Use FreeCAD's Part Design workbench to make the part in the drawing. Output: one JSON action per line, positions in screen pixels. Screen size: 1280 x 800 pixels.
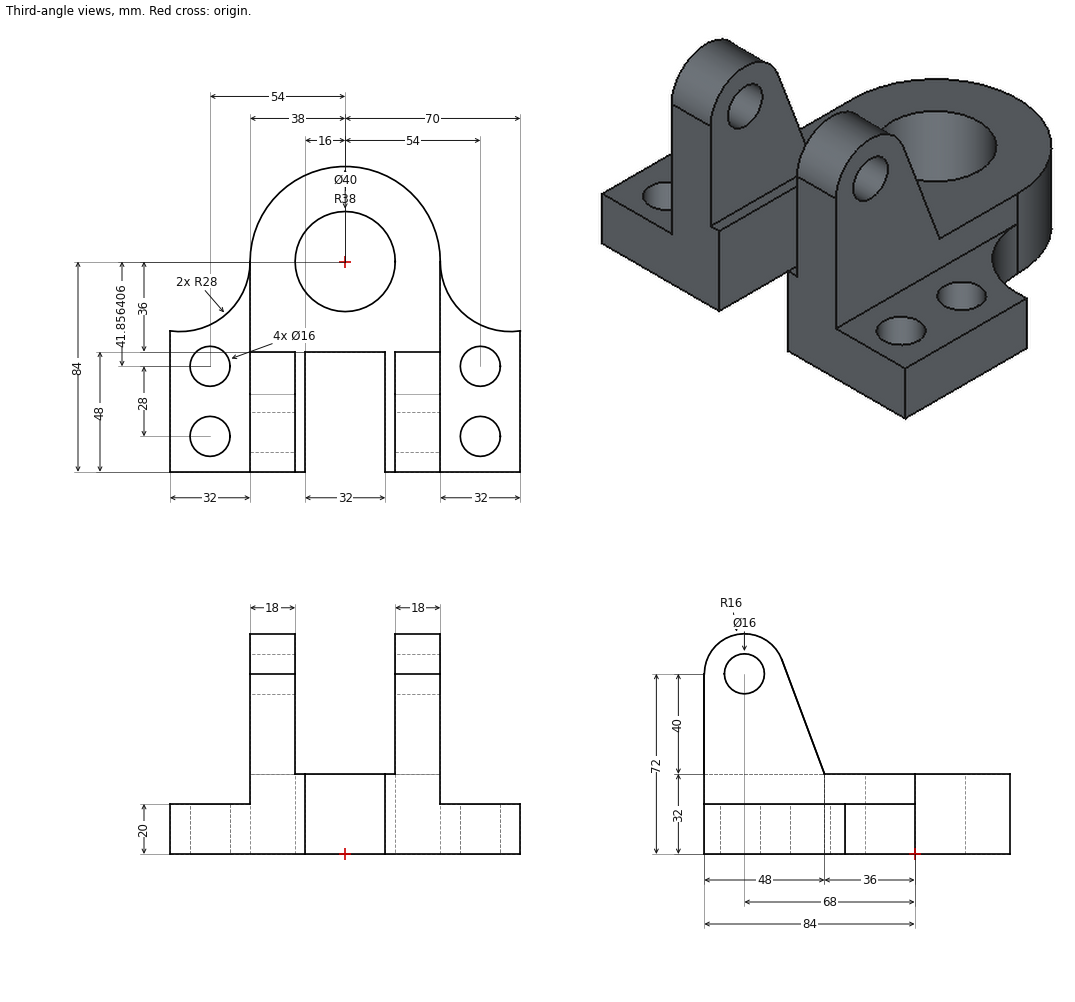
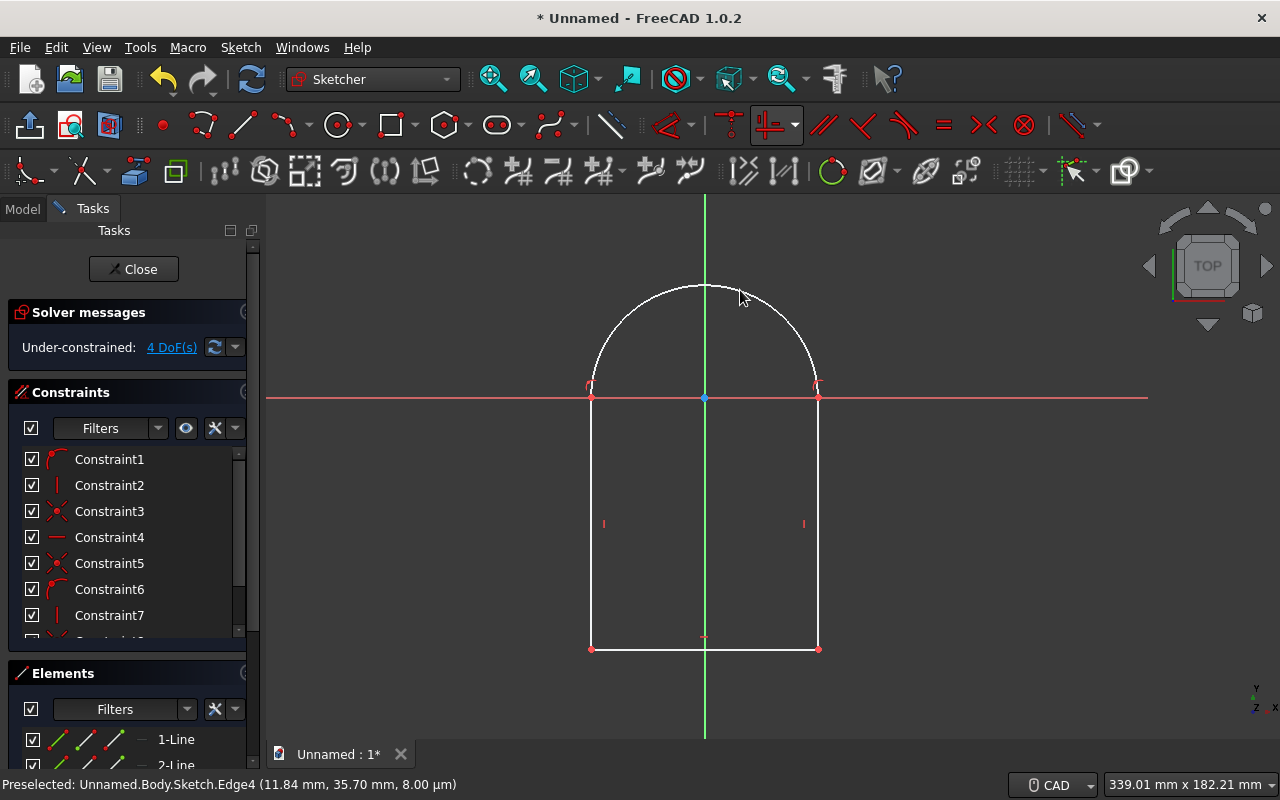
{"action": "left_click_drag", "start_coordinate": [695, 388], "coordinate": [715, 409]}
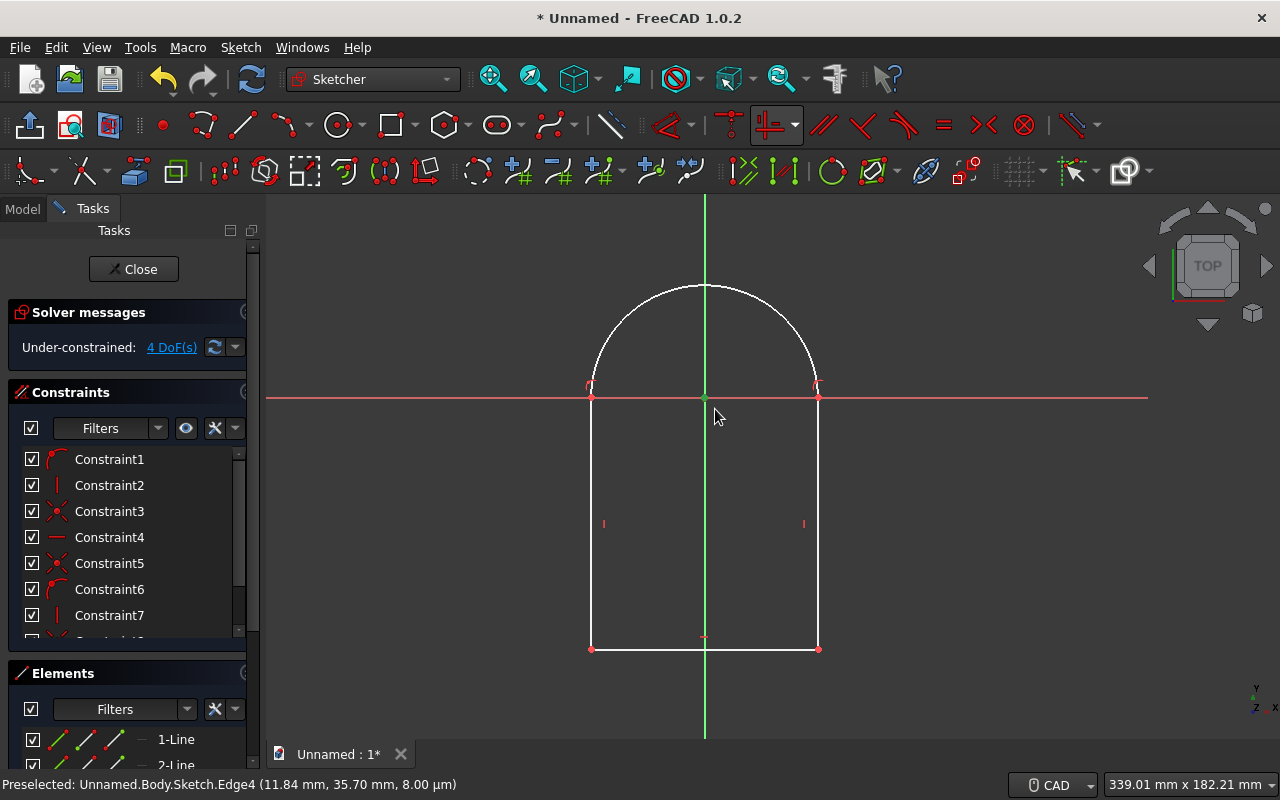
{"action": "left_click", "coordinate": [730, 126]}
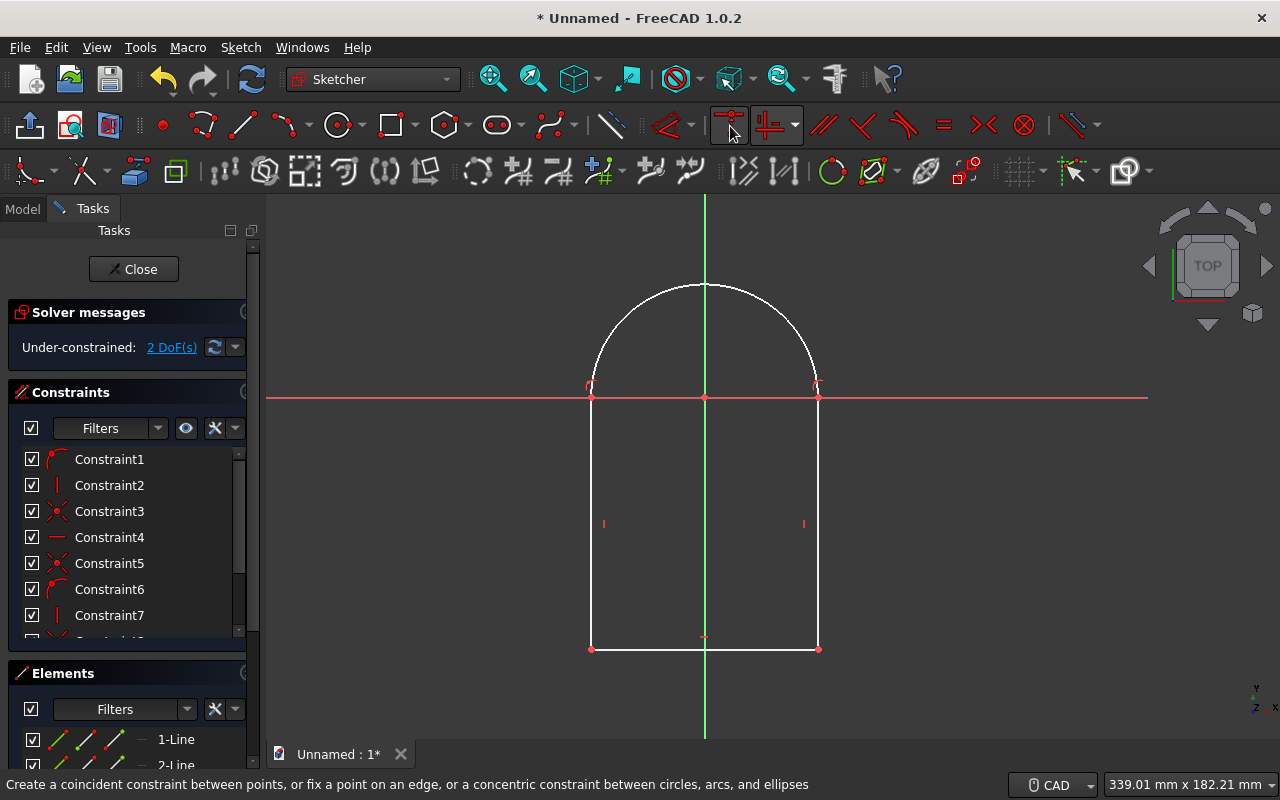
{"action": "left_click", "coordinate": [666, 126]}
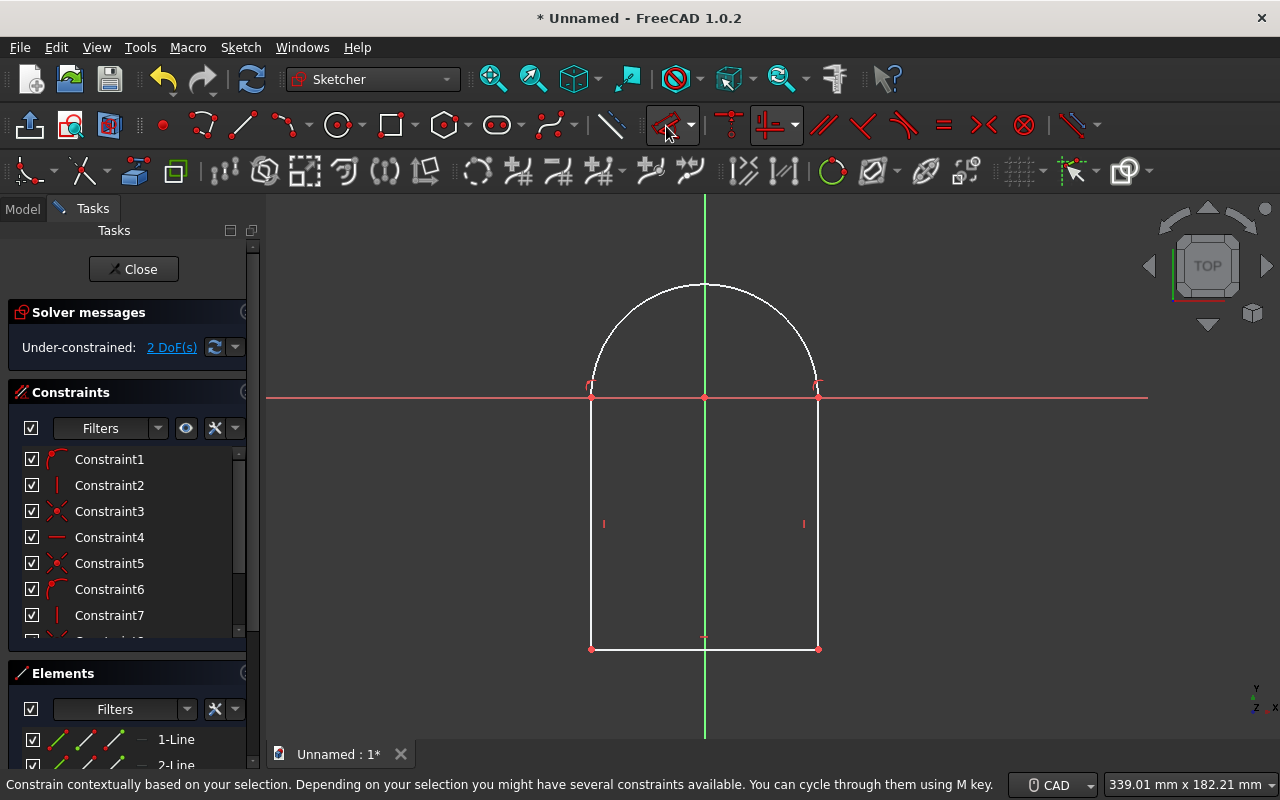
{"action": "left_click", "coordinate": [771, 306]}
{"action": "left_click", "coordinate": [790, 280]}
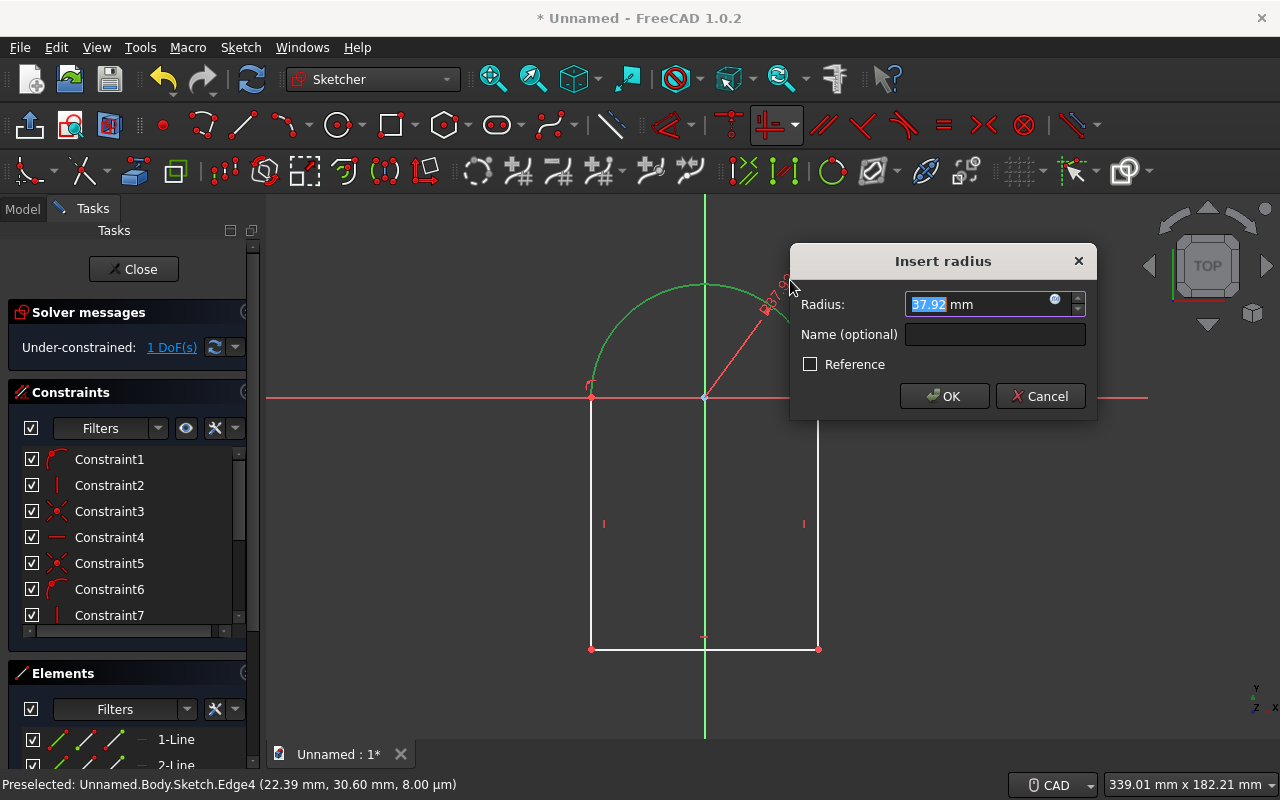
{"action": "type", "text": "38"}
{"action": "key", "text": "Return"}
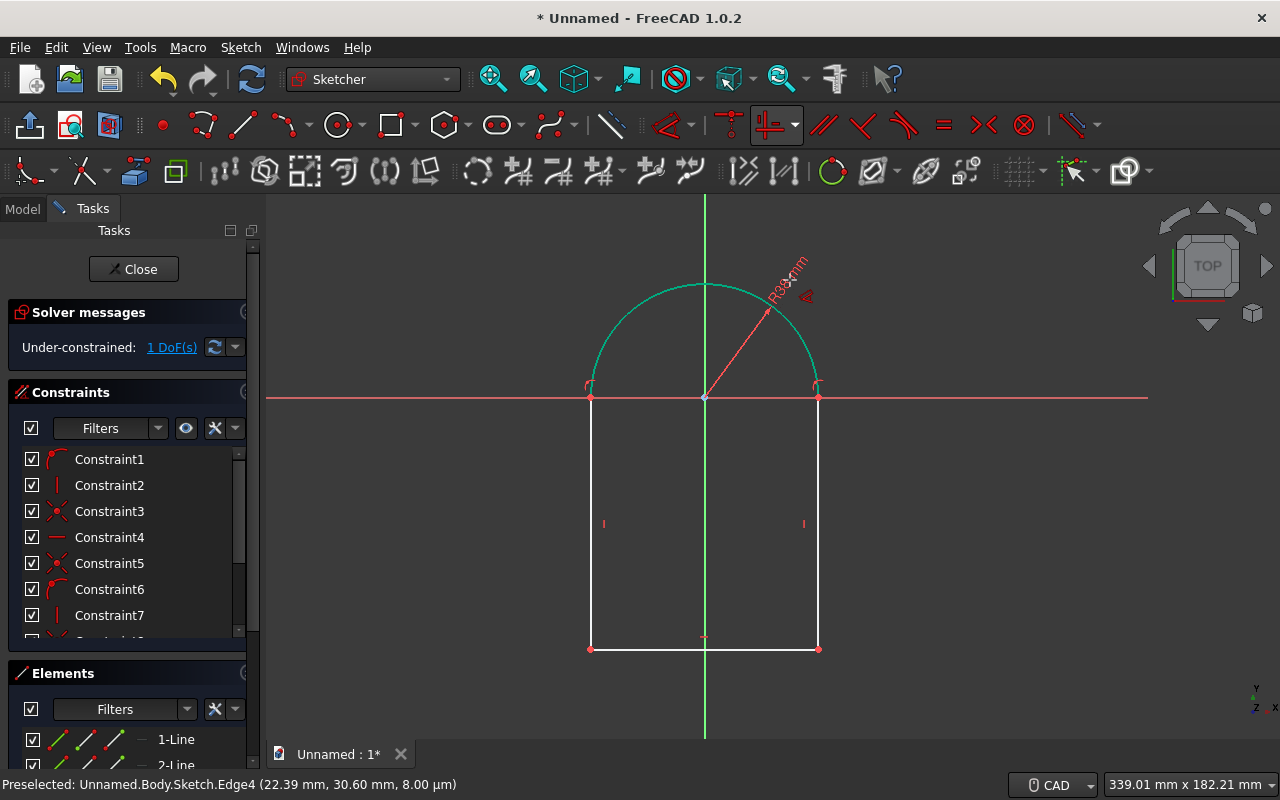
{"action": "left_click", "coordinate": [591, 473]}
{"action": "left_click", "coordinate": [557, 524]}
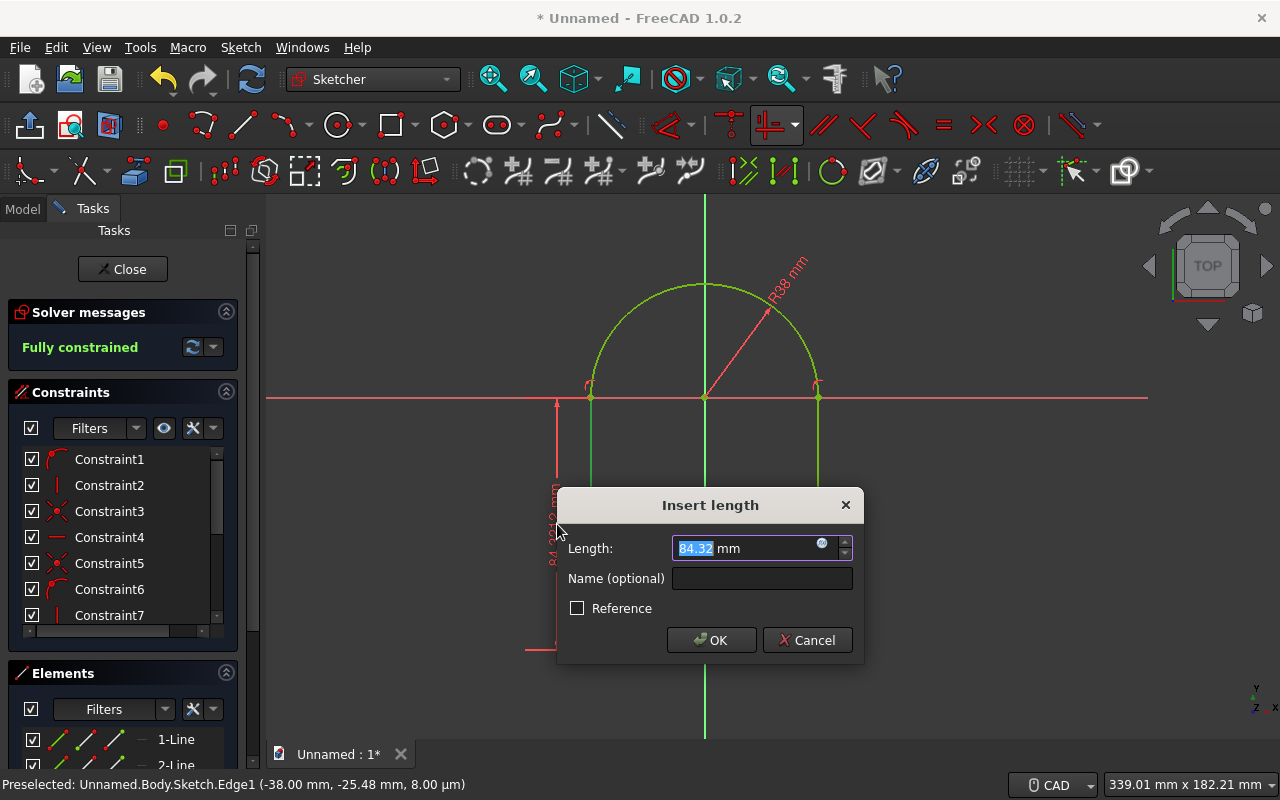
{"action": "type", "text": "84"}
{"action": "key", "text": "Return"}
{"action": "key", "text": "Escape"}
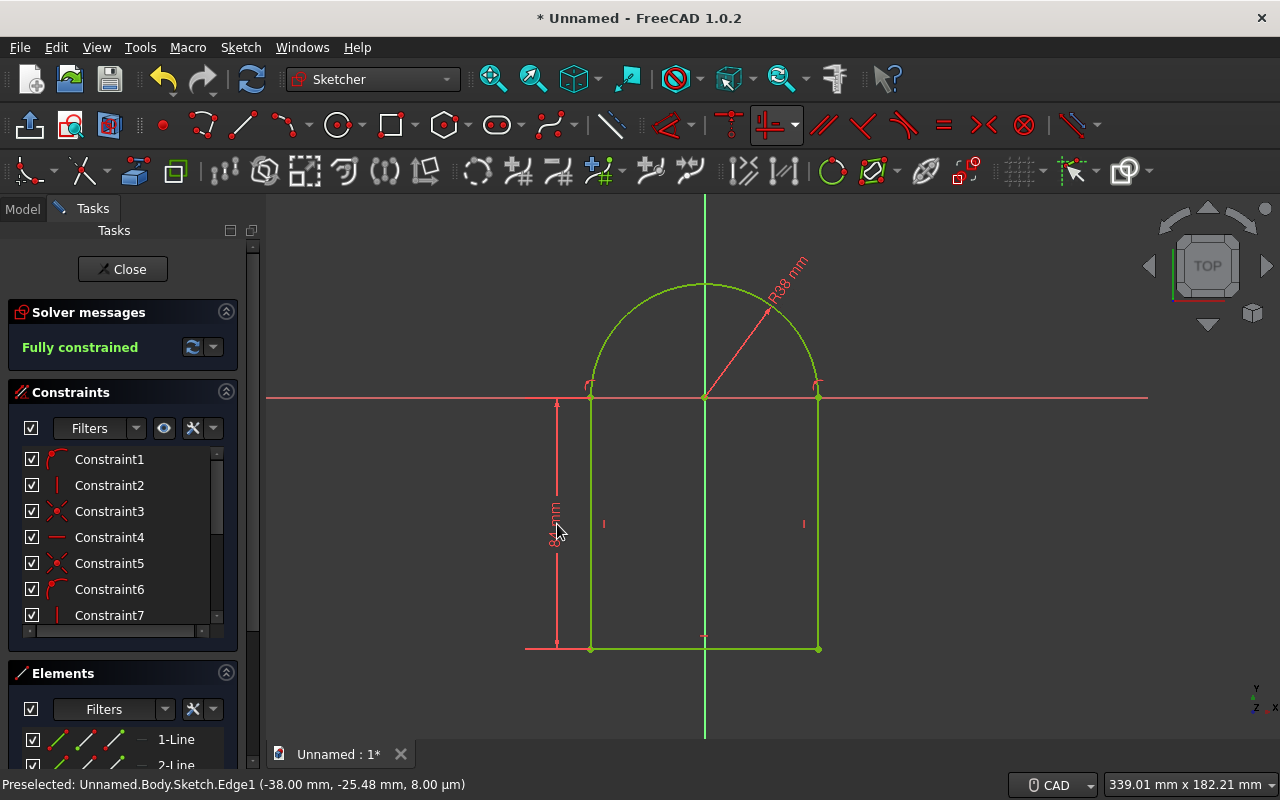
{"action": "left_click", "coordinate": [123, 269]}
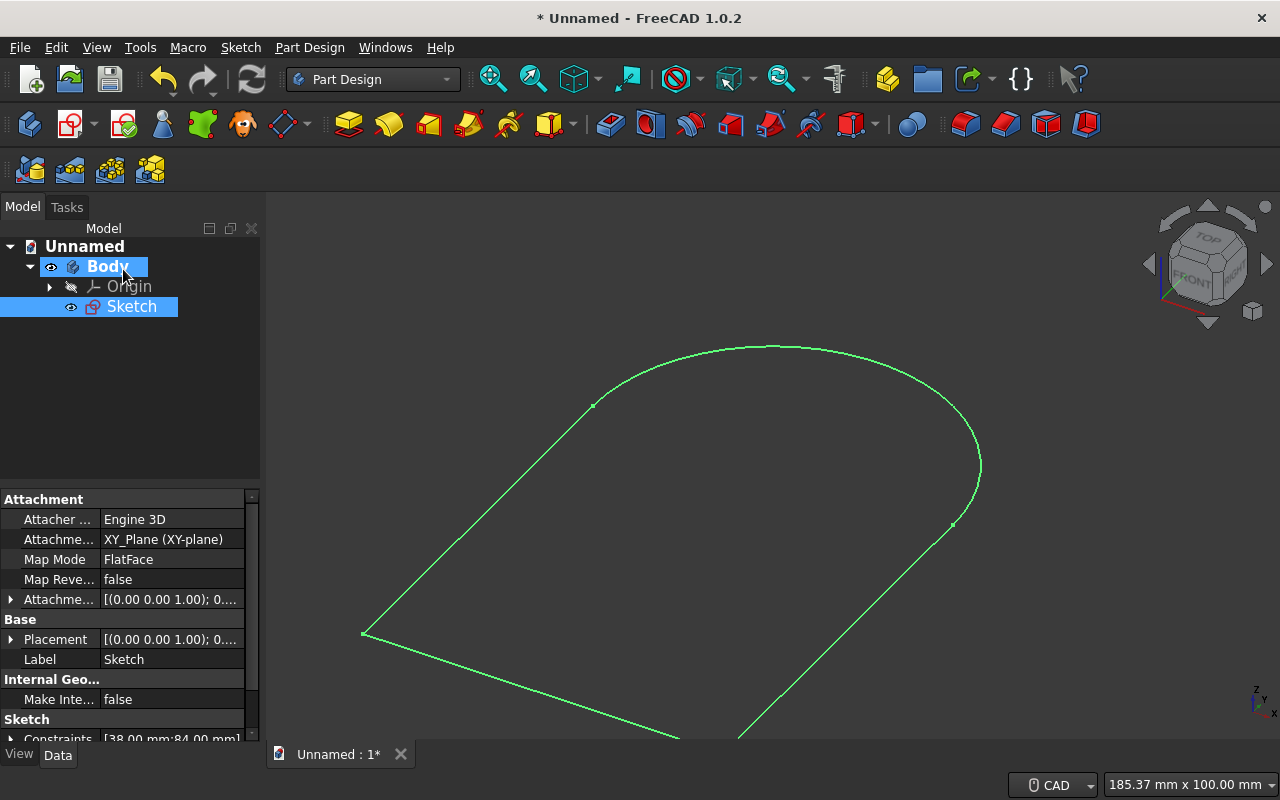
{"action": "left_click", "coordinate": [350, 124]}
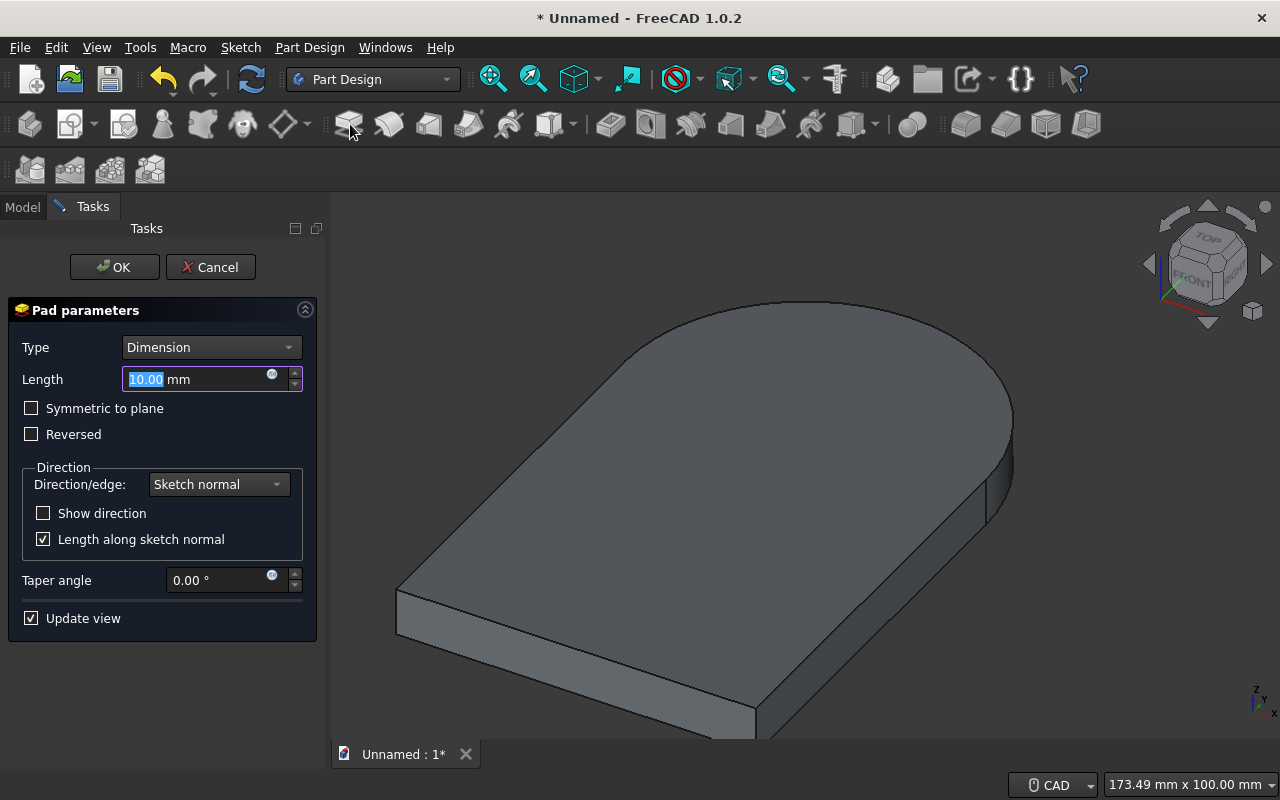
{"action": "type", "text": "32"}
{"action": "key", "text": "Tab"}